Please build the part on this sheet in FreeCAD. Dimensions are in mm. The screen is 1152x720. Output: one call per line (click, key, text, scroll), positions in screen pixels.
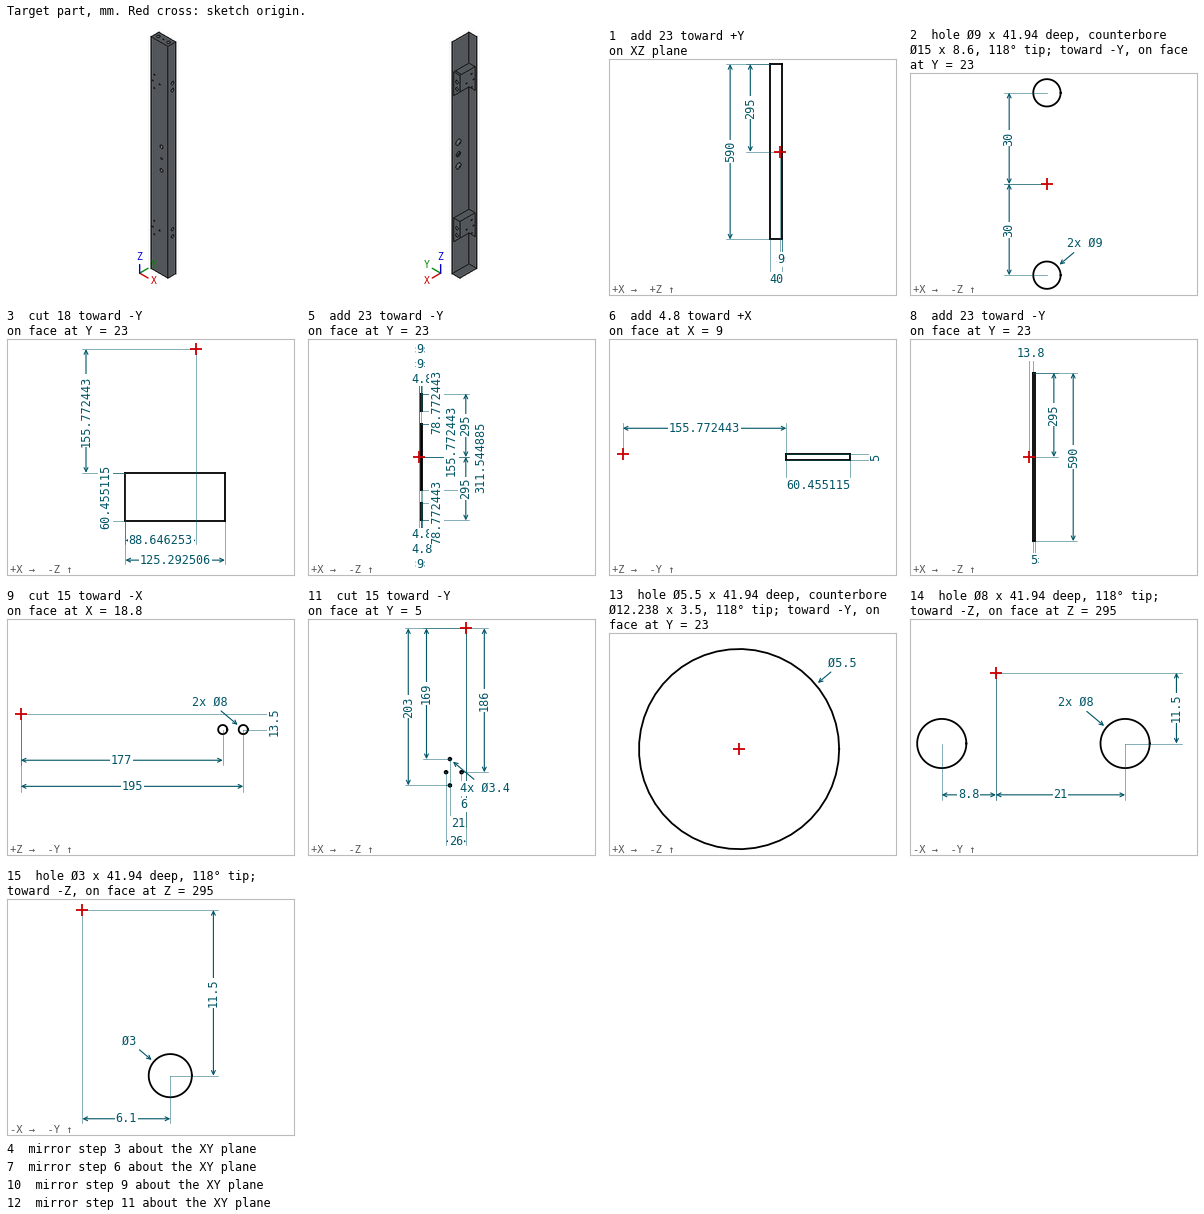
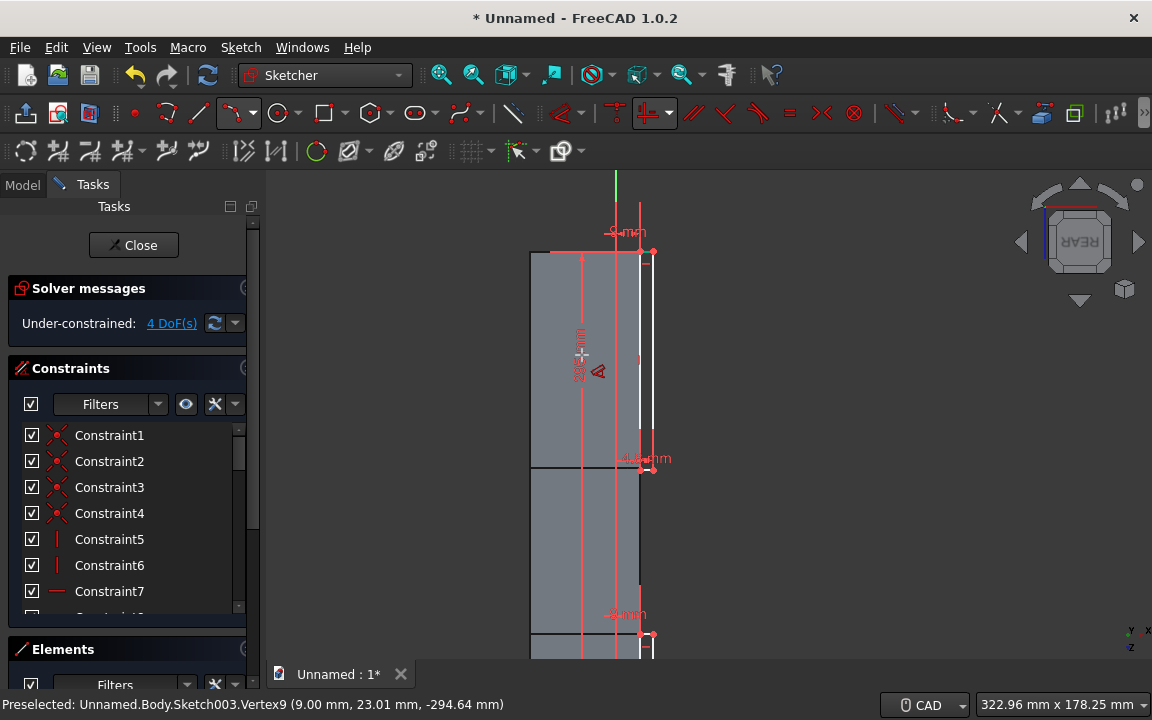
scroll(642, 251, down, 8)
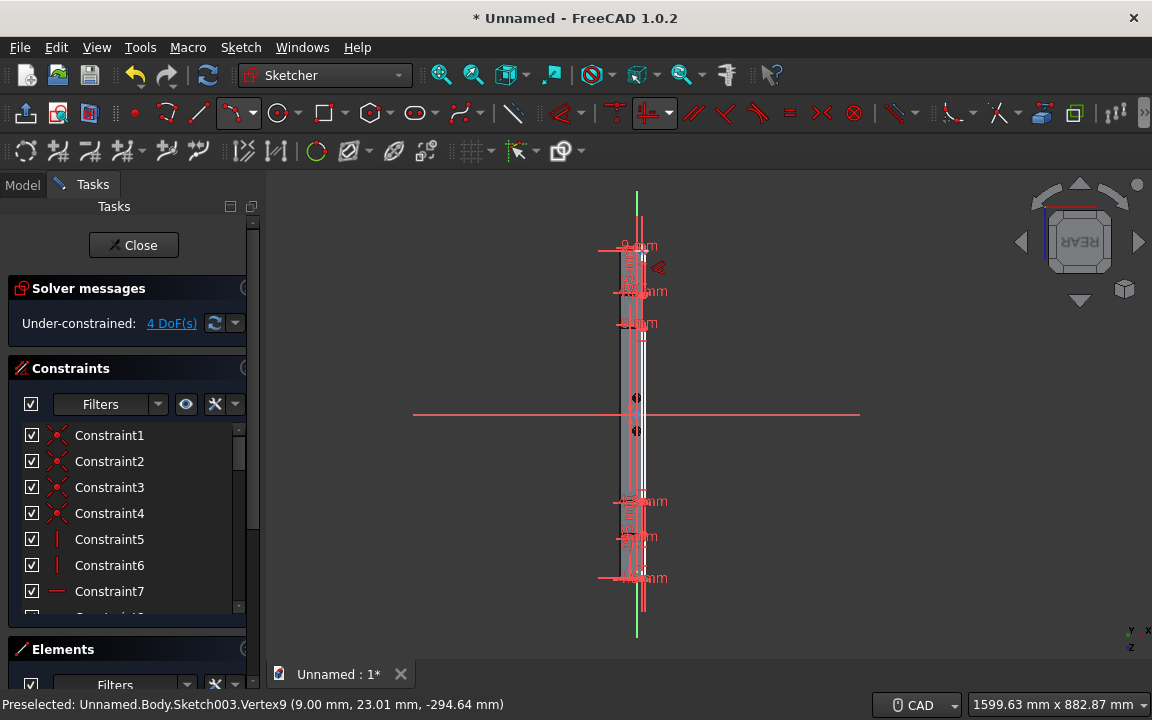
scroll(642, 548, up, 9)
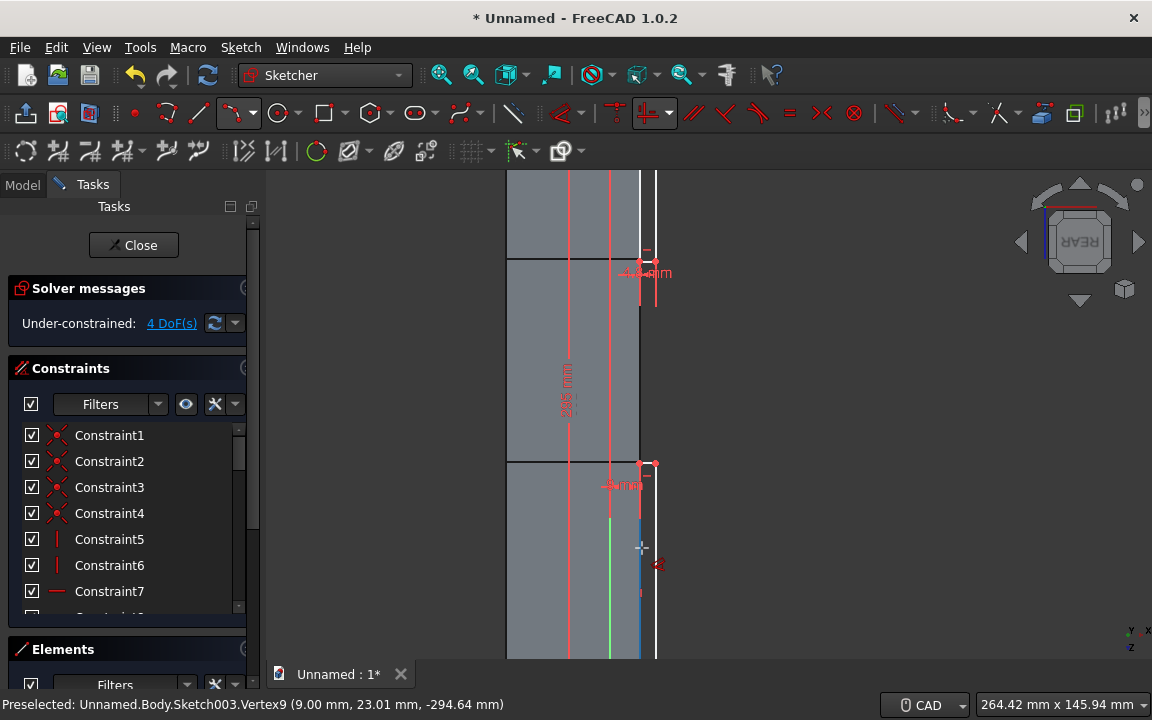
click(640, 542)
click(674, 547)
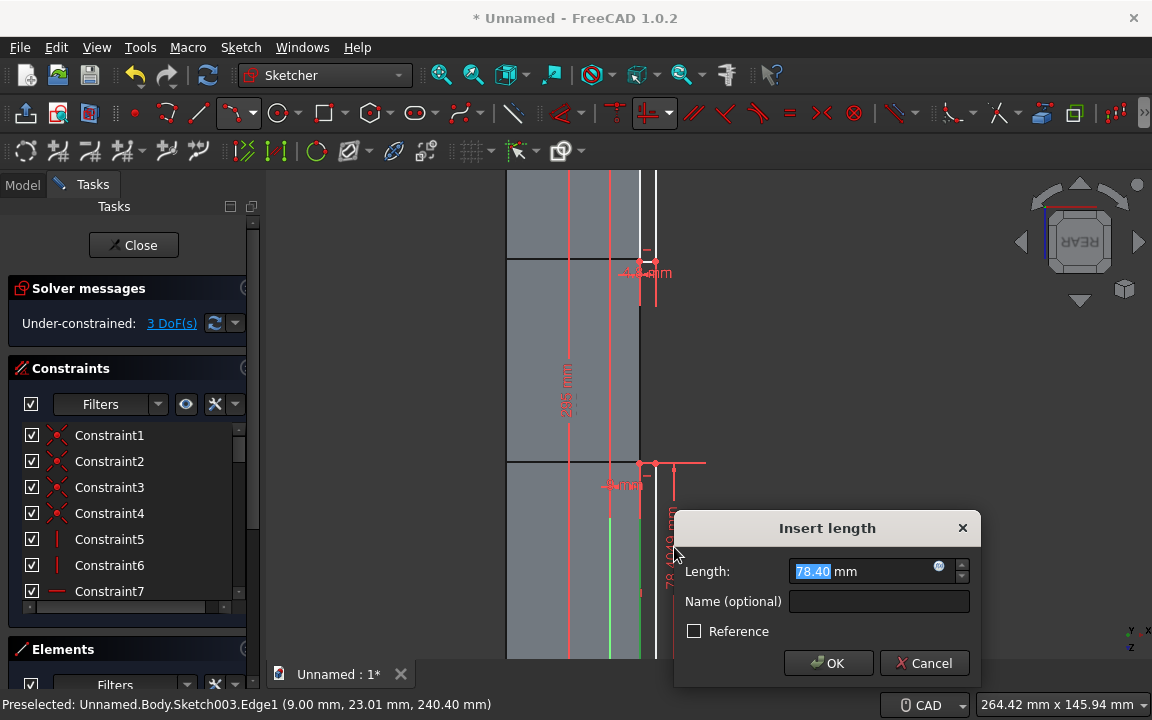
text(78.772443)
key(Return)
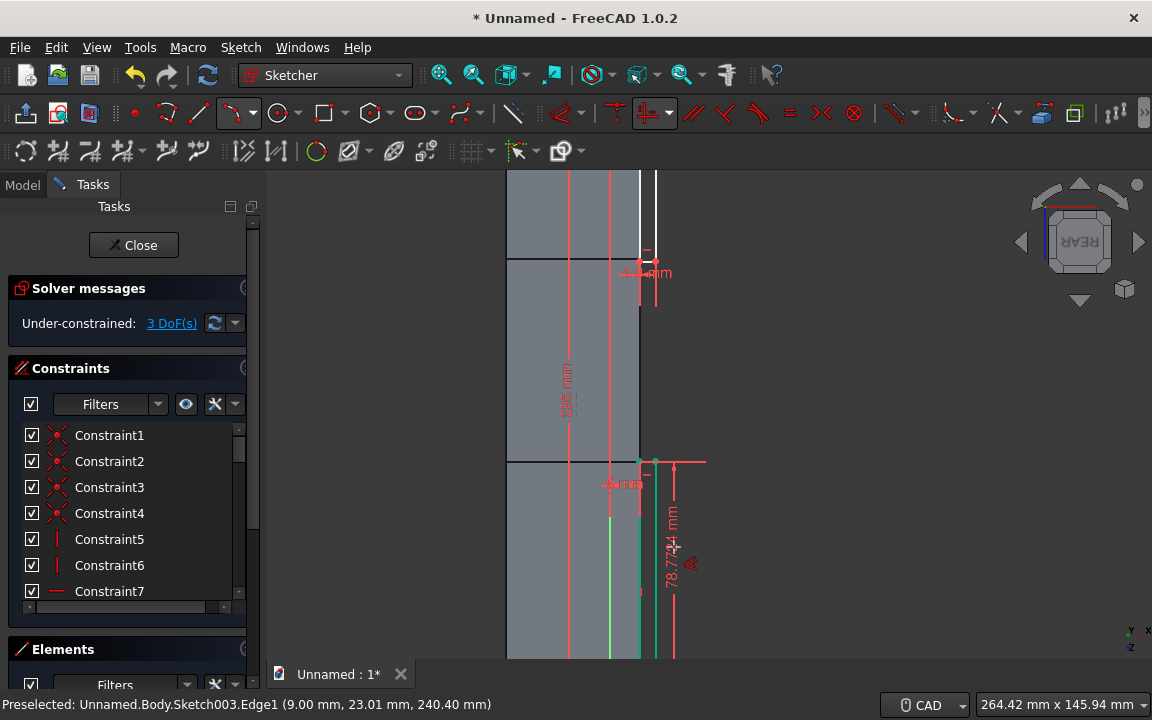
scroll(642, 549, down, 9)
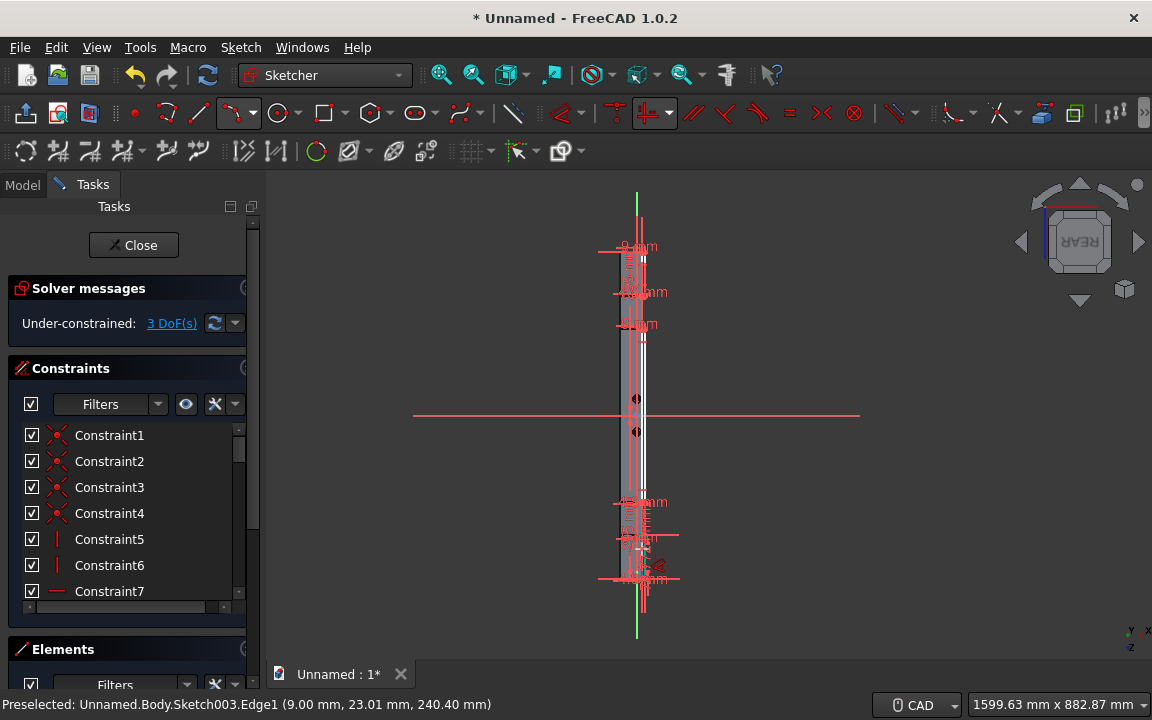
scroll(642, 265, up, 9)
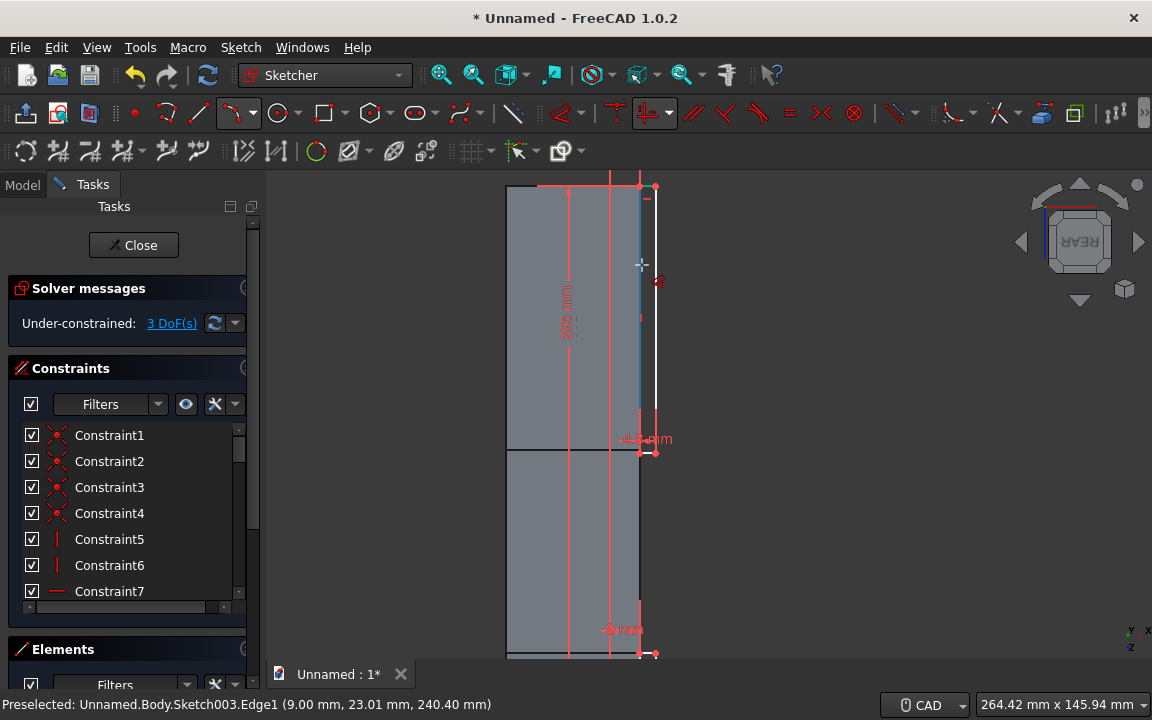
click(640, 266)
click(674, 326)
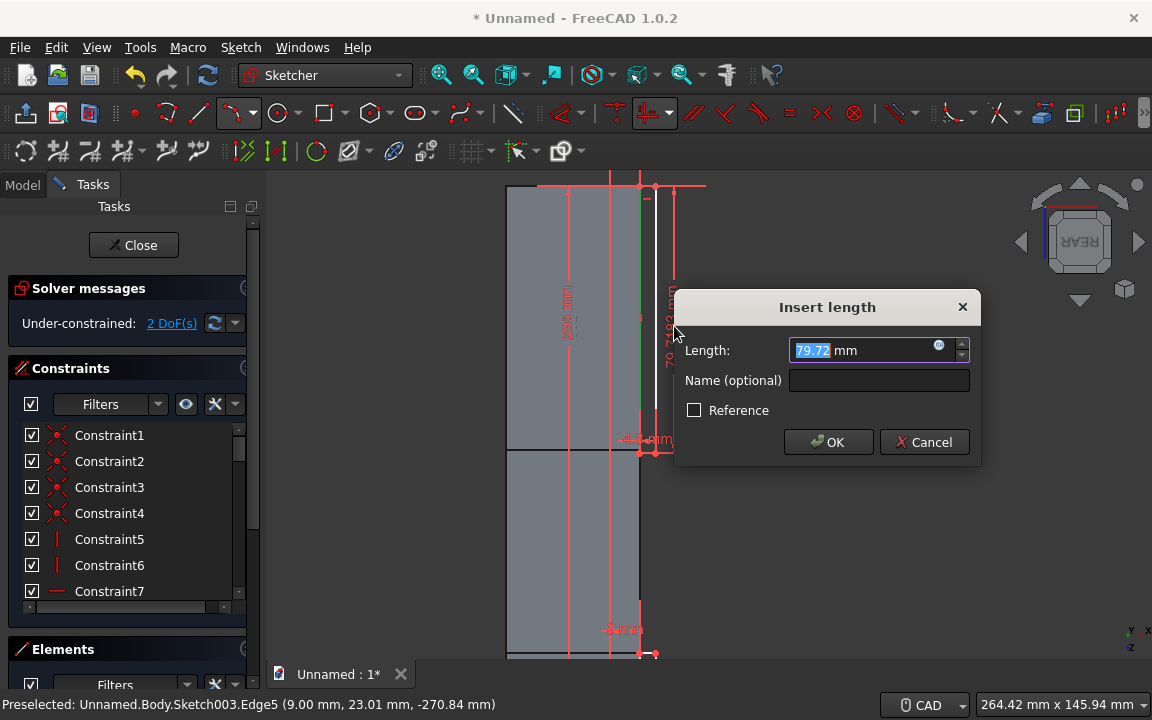
text(78.772443)
key(Return)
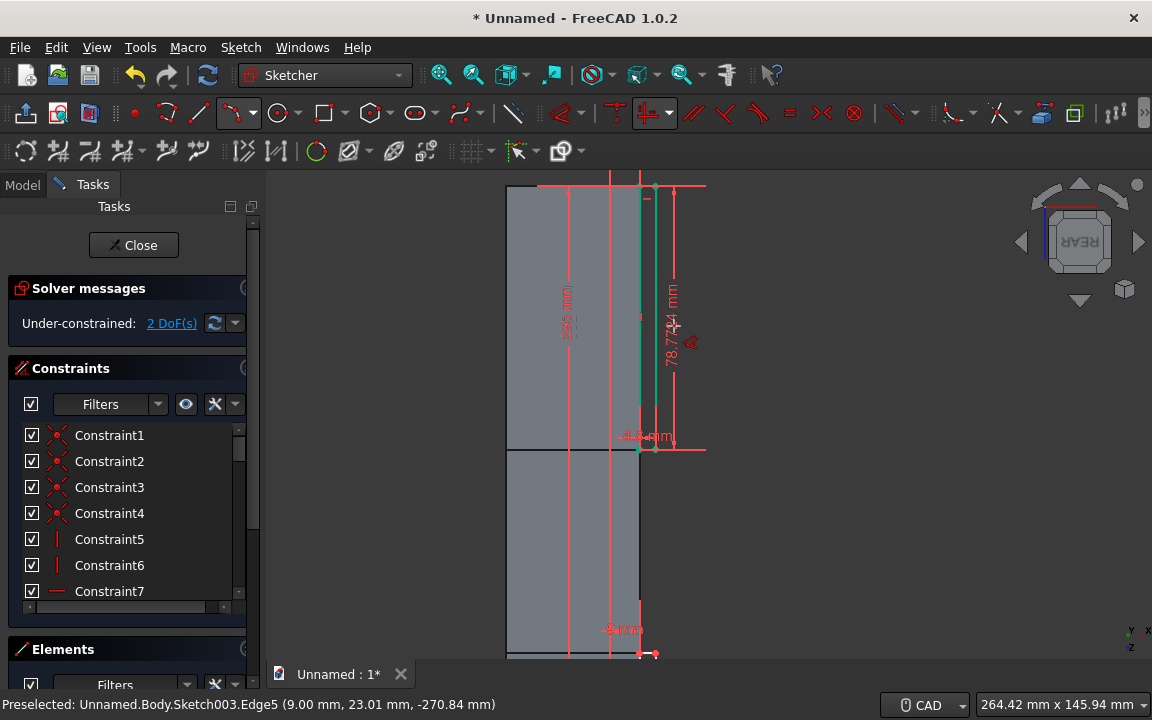
scroll(642, 264, down, 9)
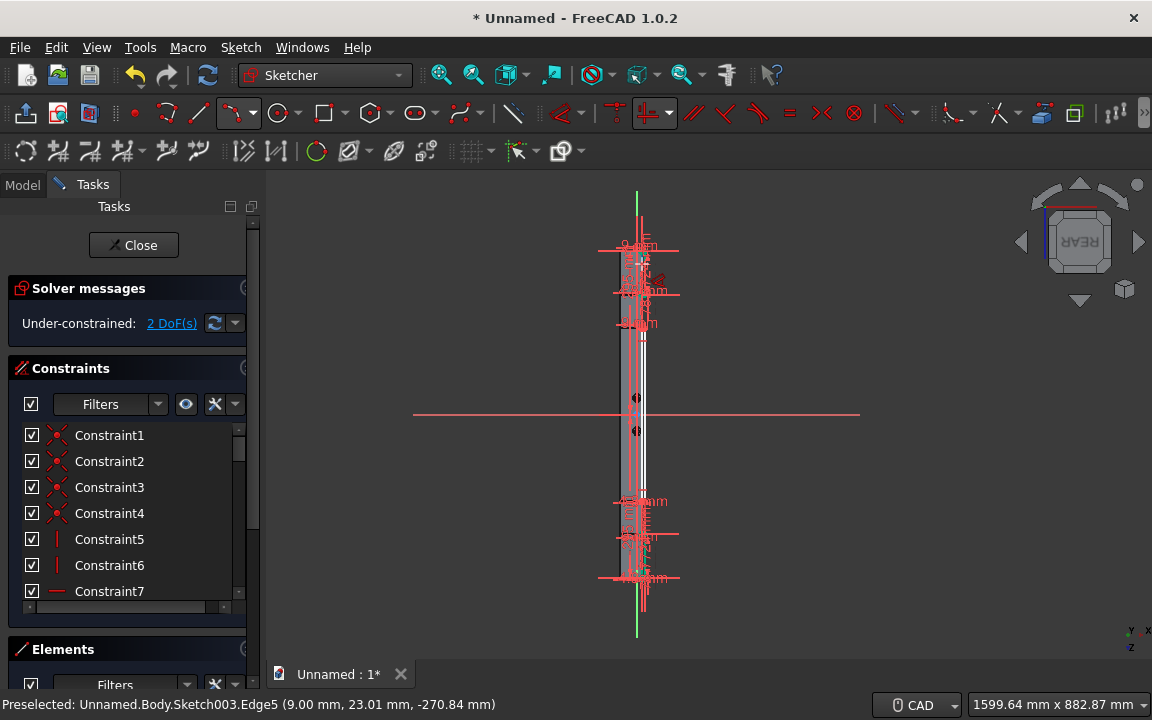
scroll(642, 380, up, 9)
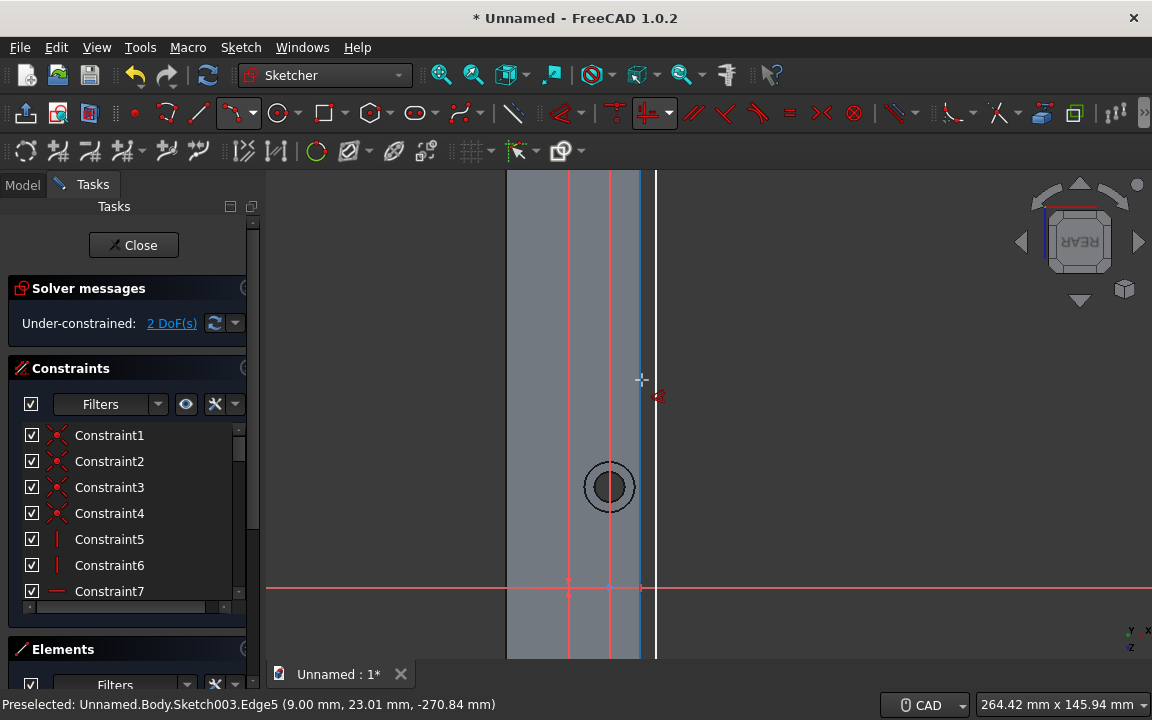
click(640, 380)
click(674, 414)